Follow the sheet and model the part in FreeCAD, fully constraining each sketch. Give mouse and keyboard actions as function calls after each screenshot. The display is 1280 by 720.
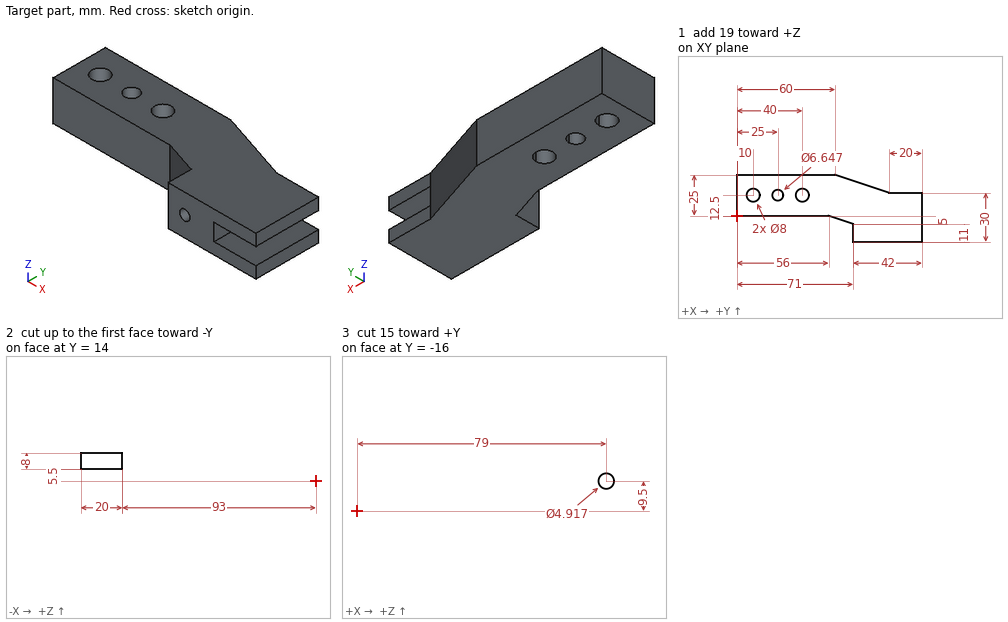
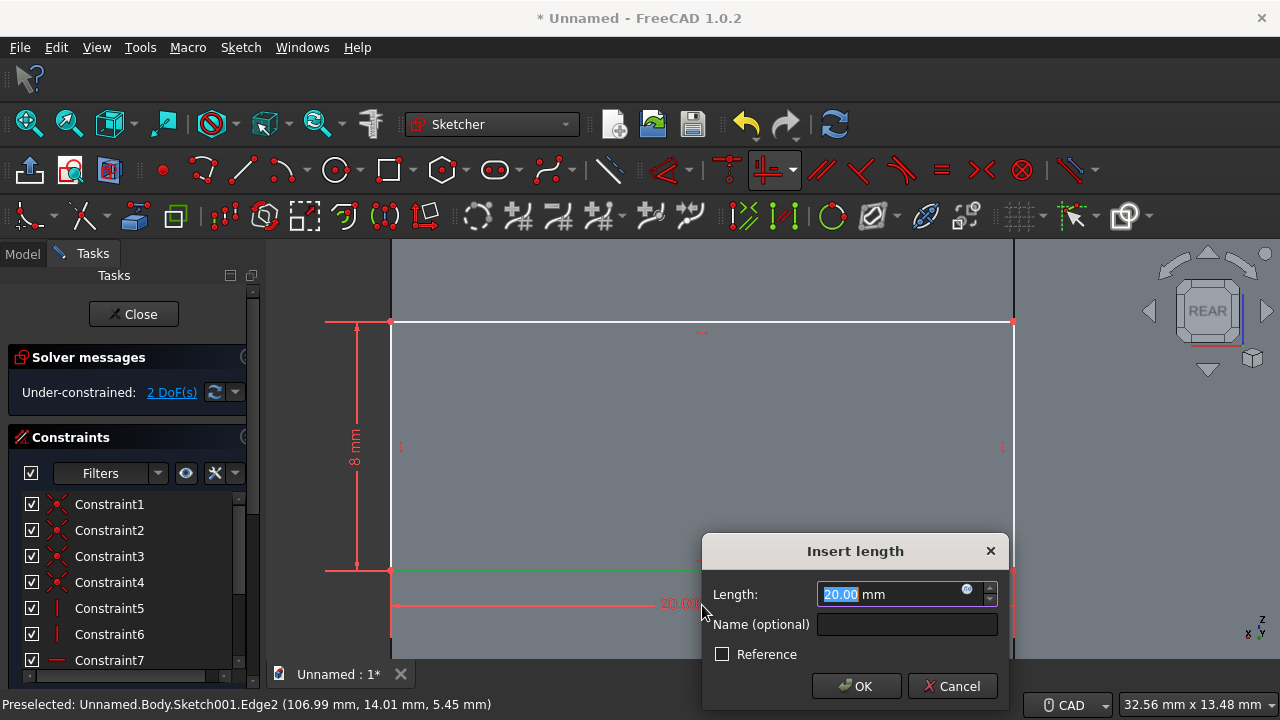
text(20)
key(Return)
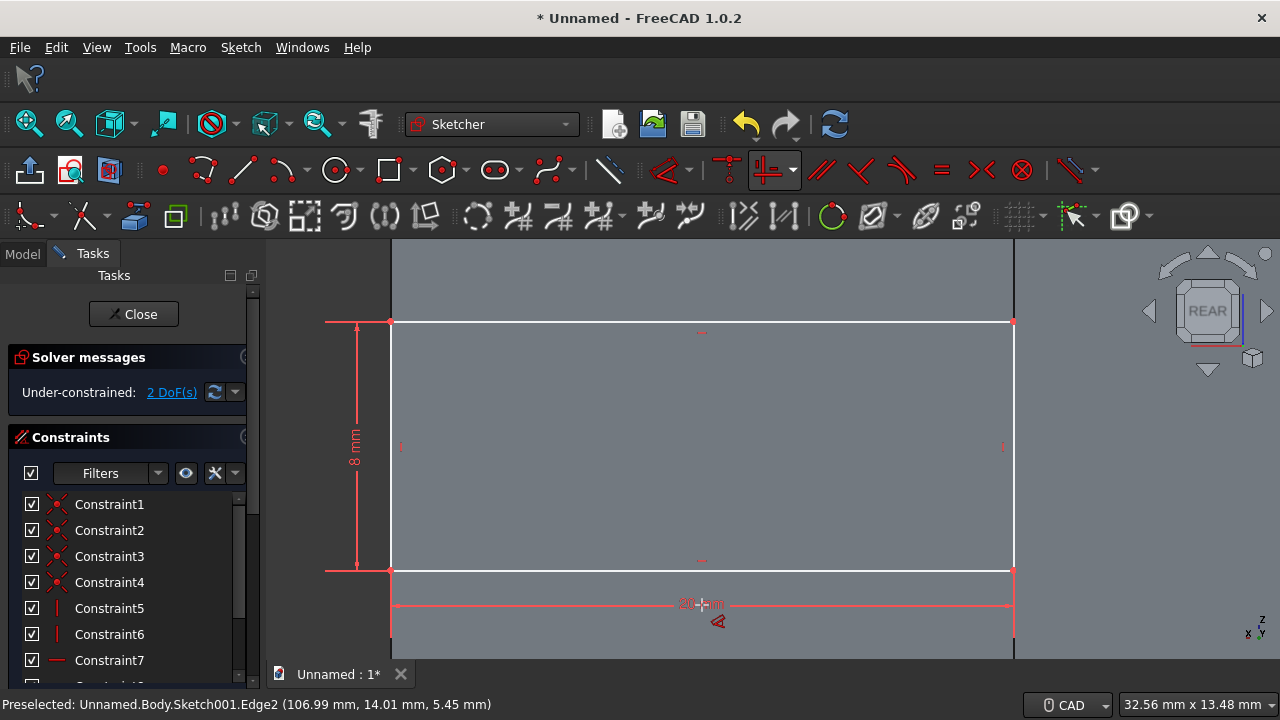
click(1014, 571)
click(1064, 537)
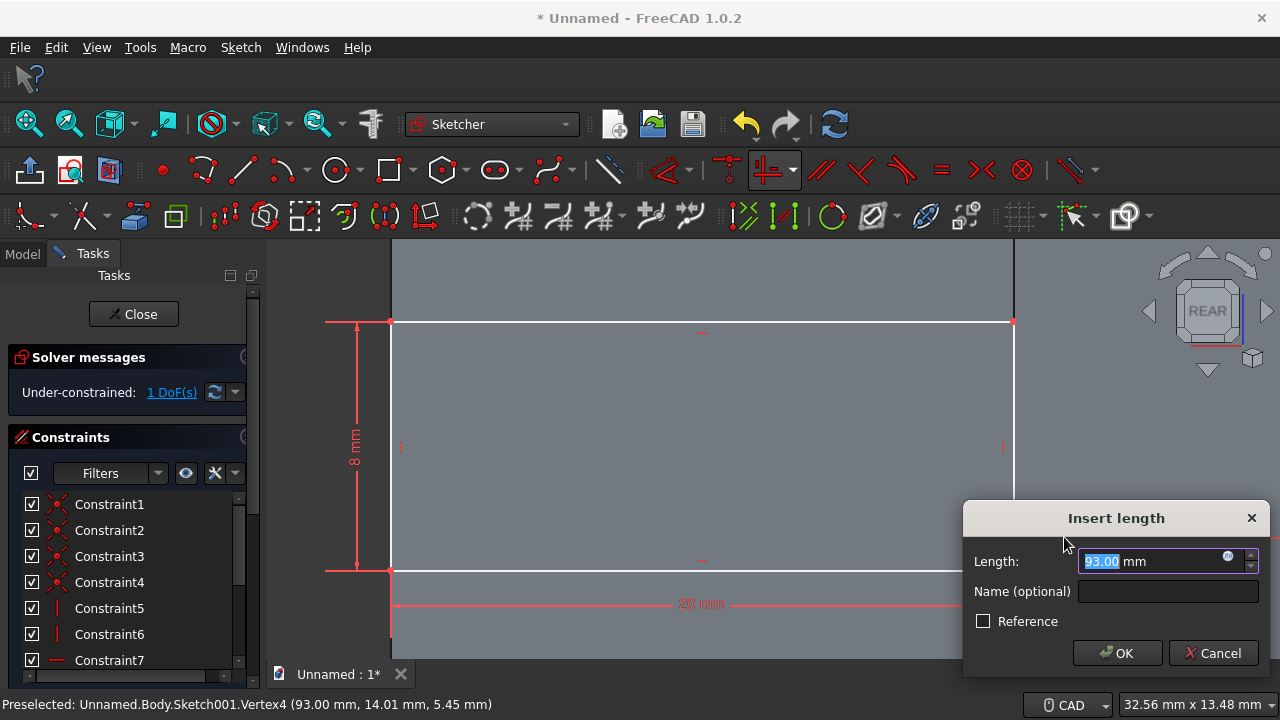
text(93)
key(Return)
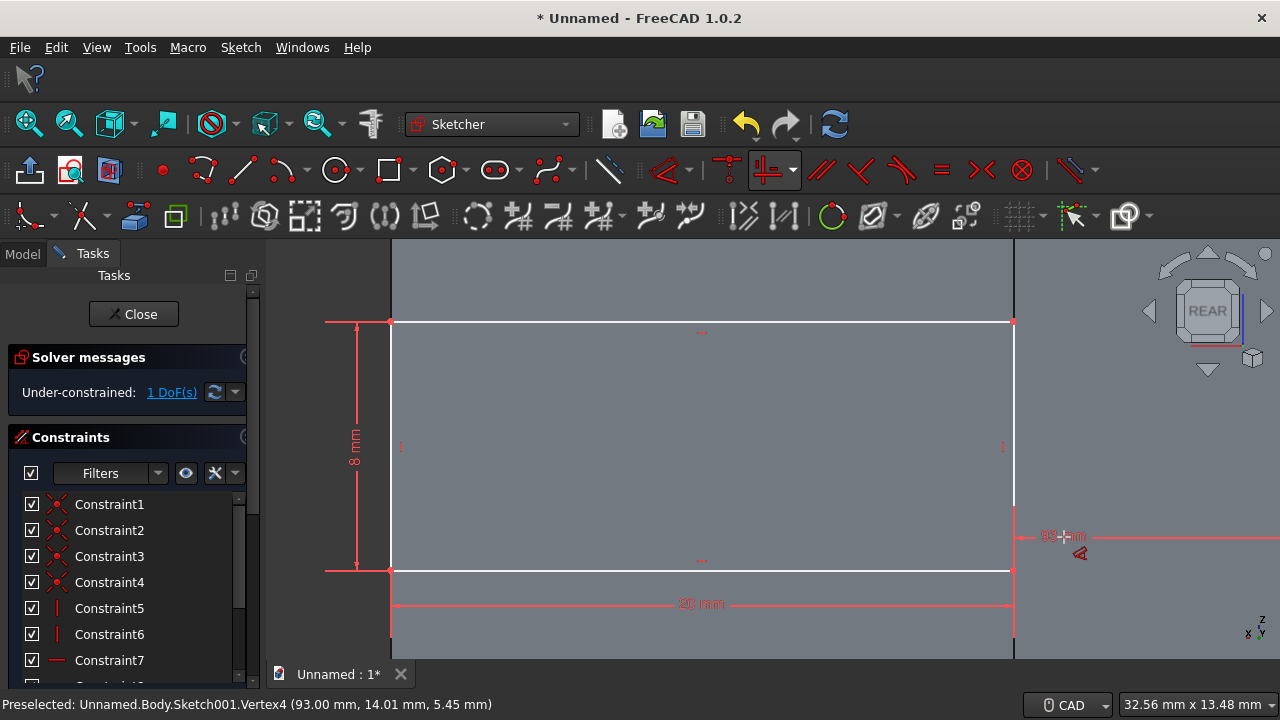
click(391, 571)
click(357, 601)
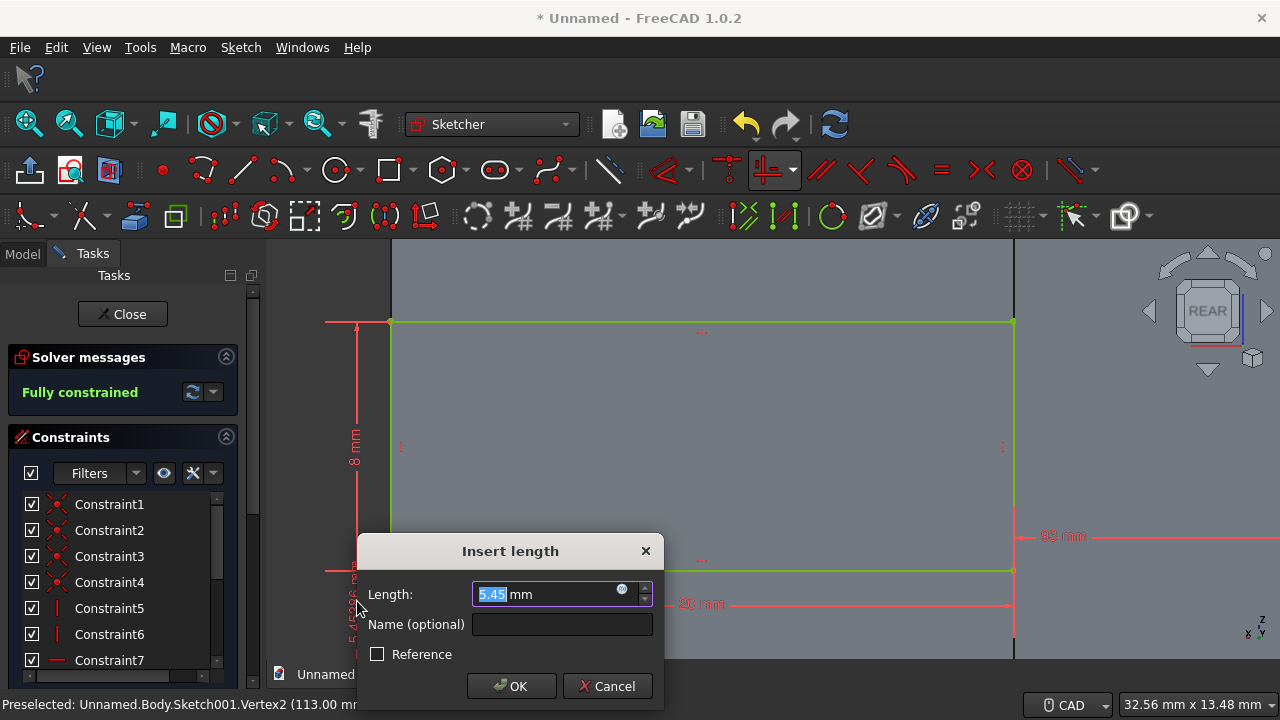
text(5.5)
key(Return)
key(Escape)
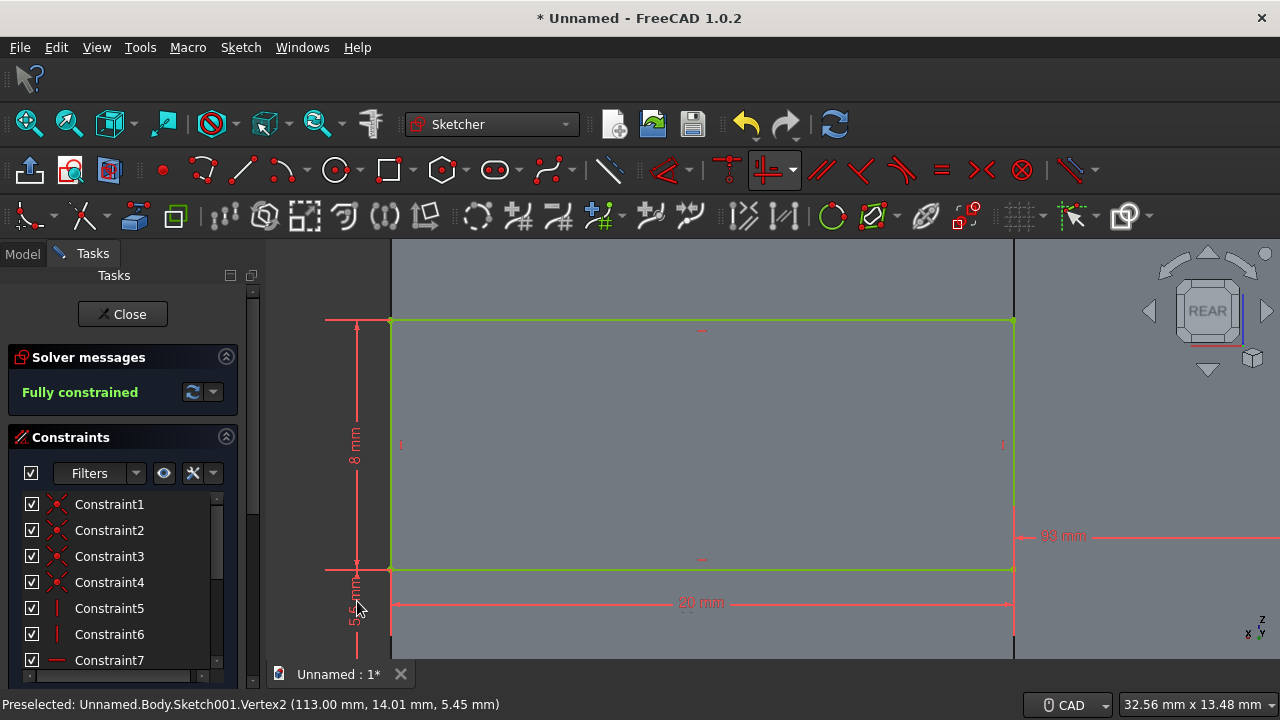
click(123, 314)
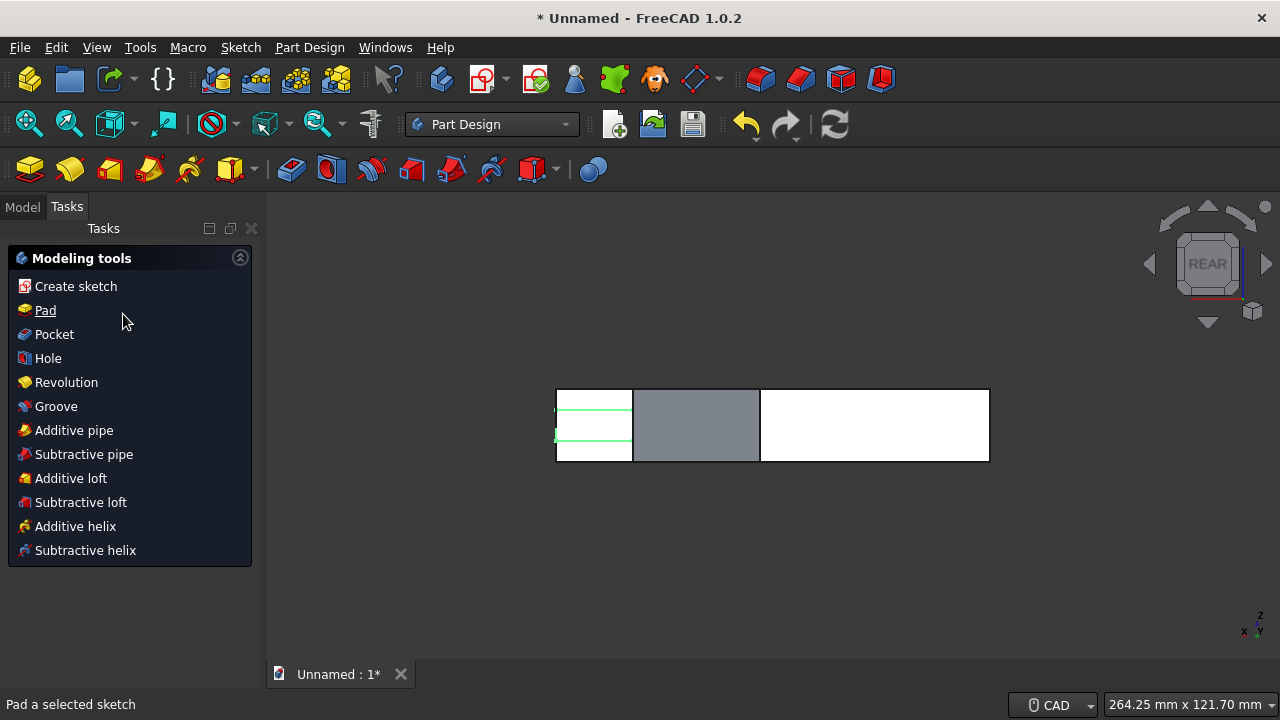
click(292, 170)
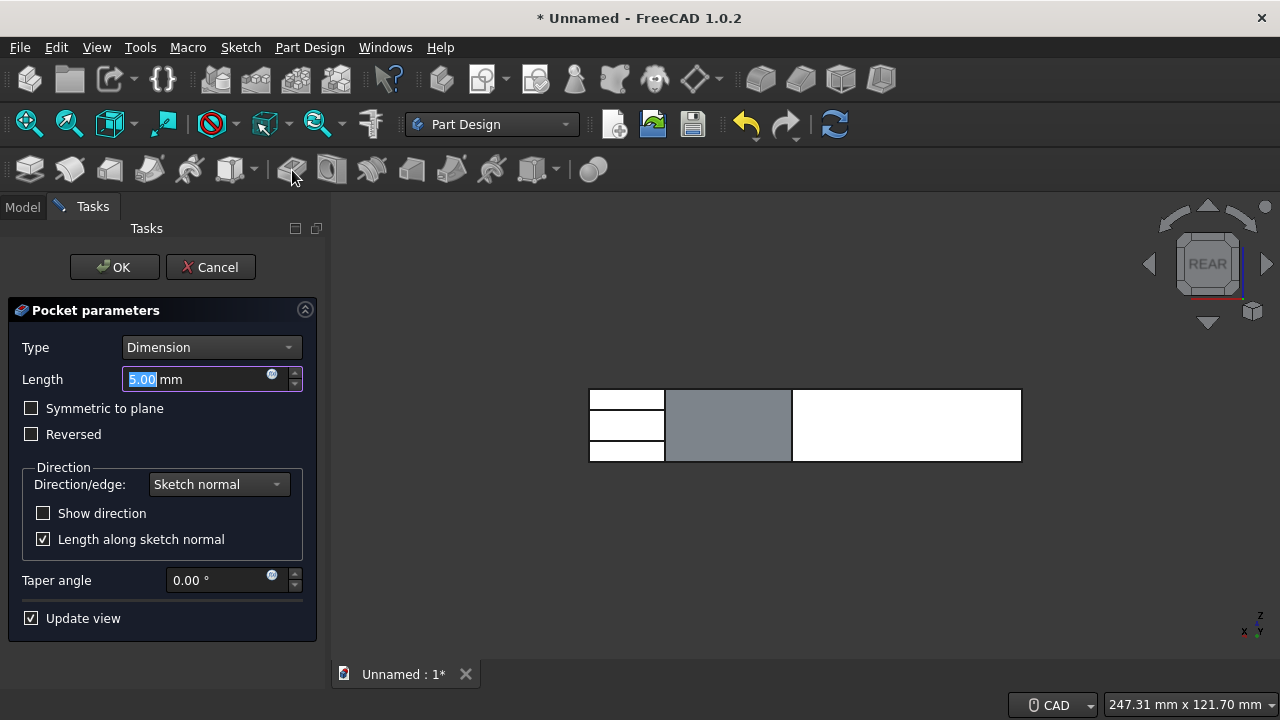
click(212, 348)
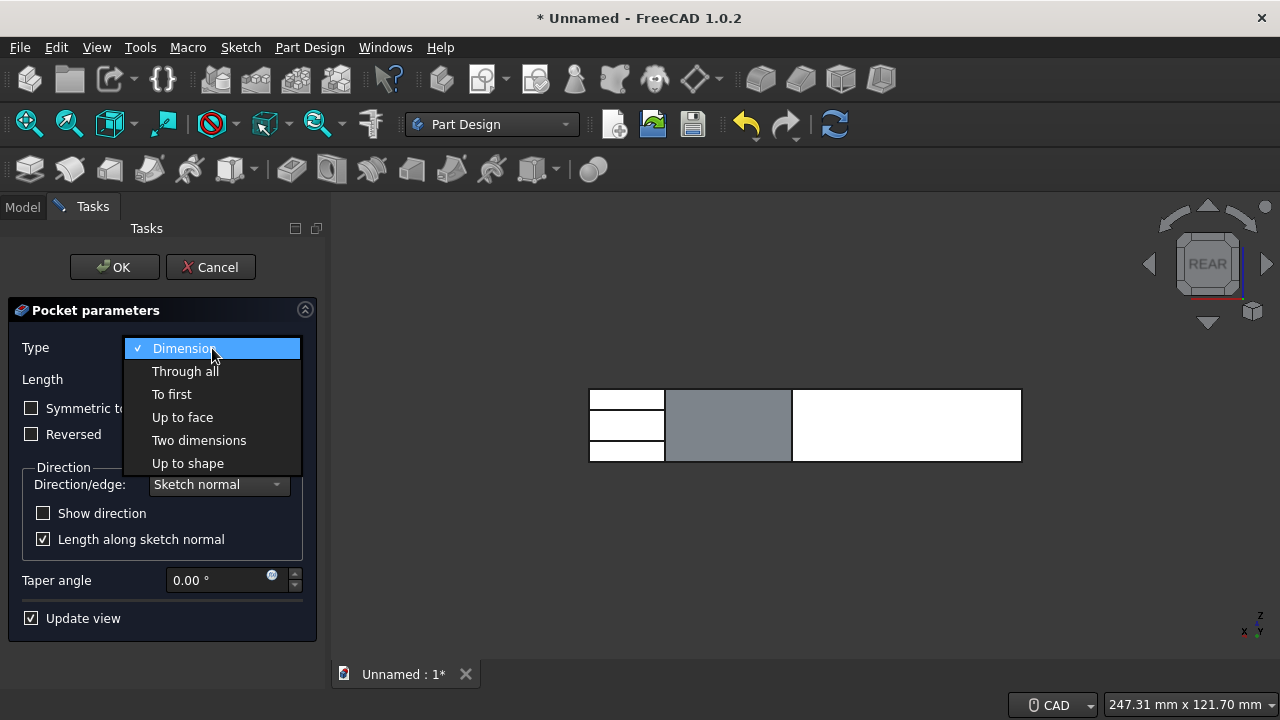
click(212, 394)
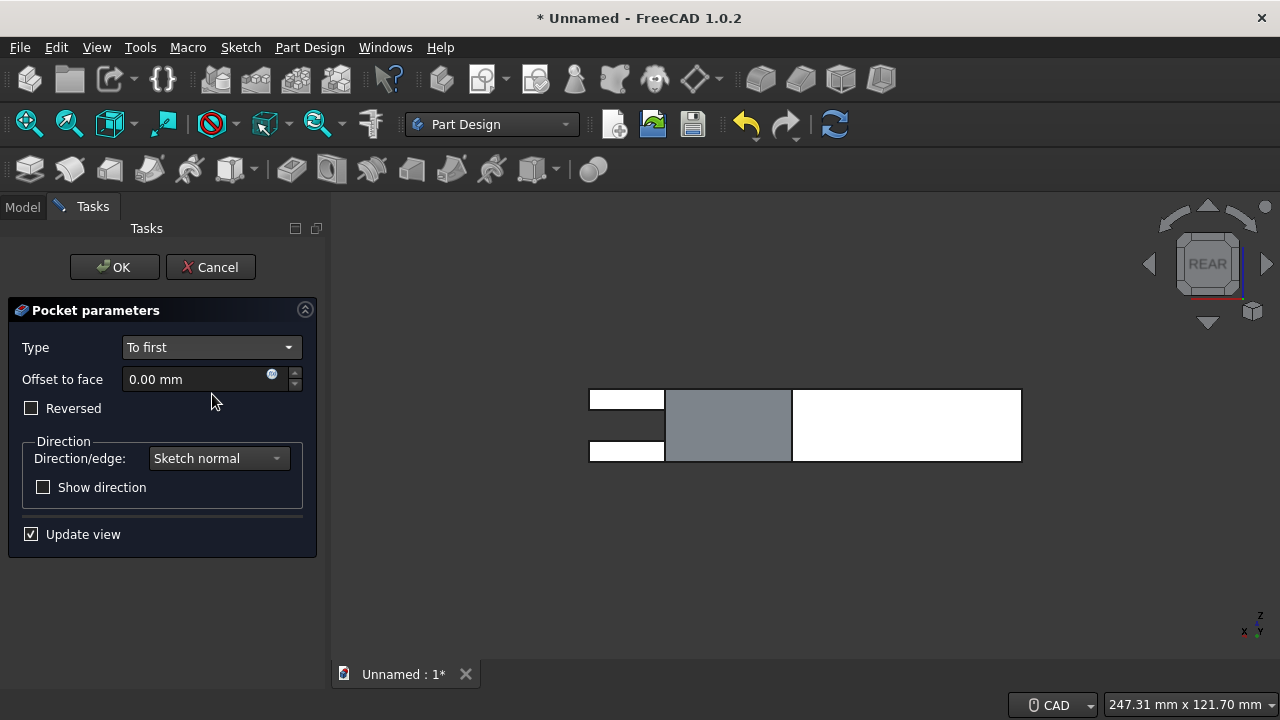
click(115, 267)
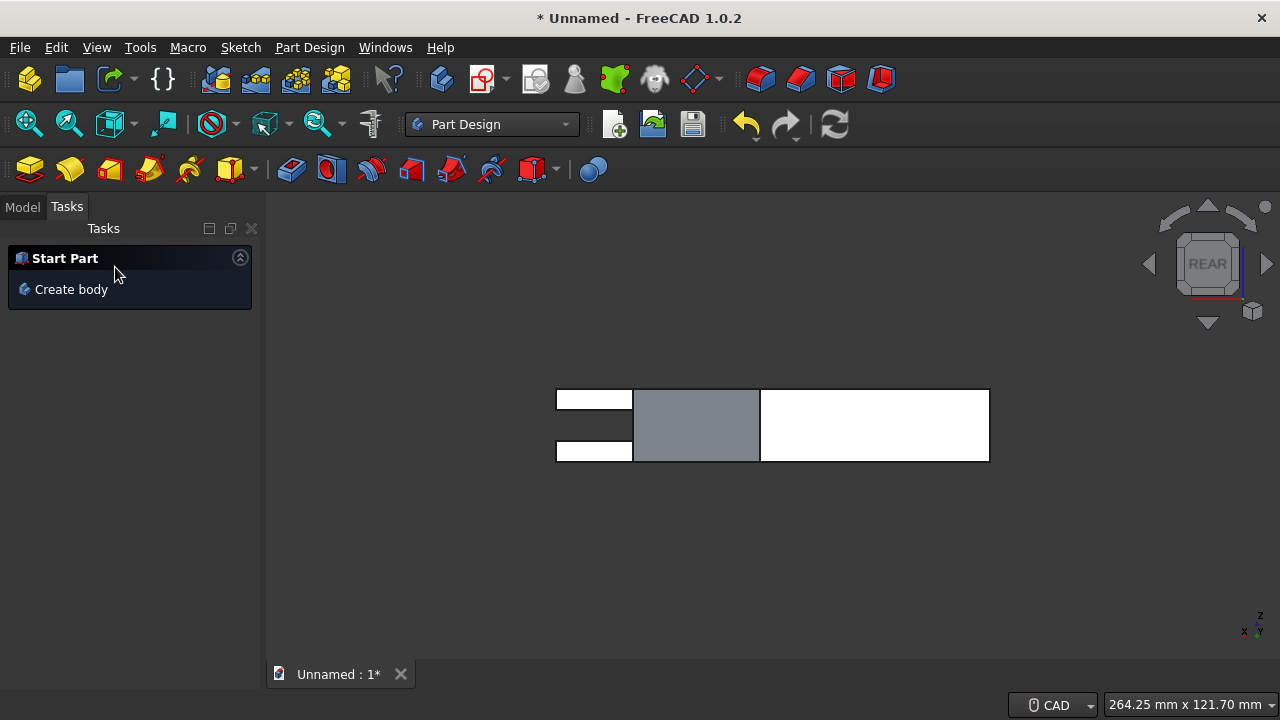
key(v)
key(f)